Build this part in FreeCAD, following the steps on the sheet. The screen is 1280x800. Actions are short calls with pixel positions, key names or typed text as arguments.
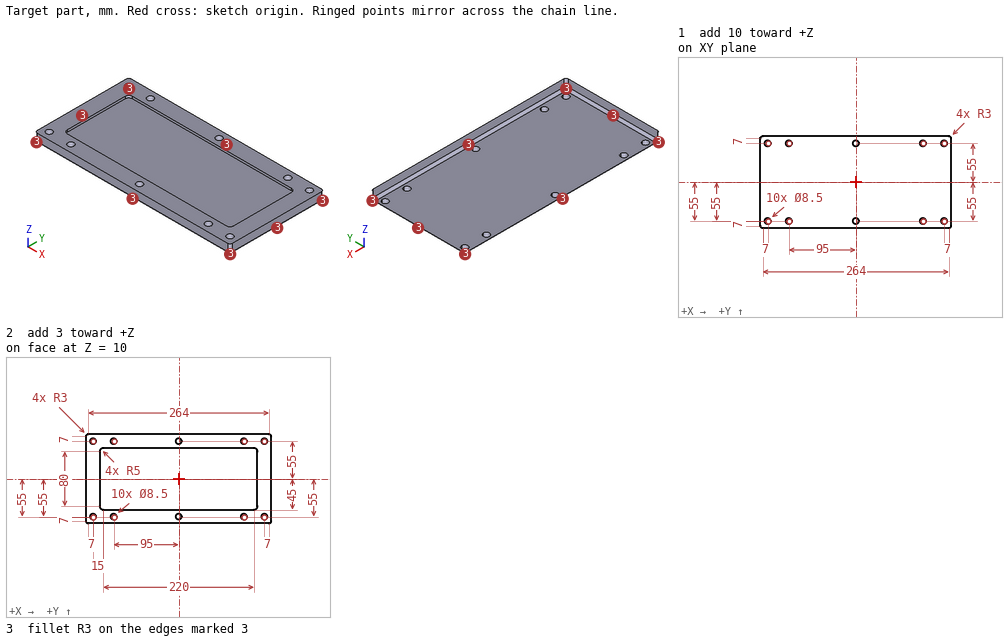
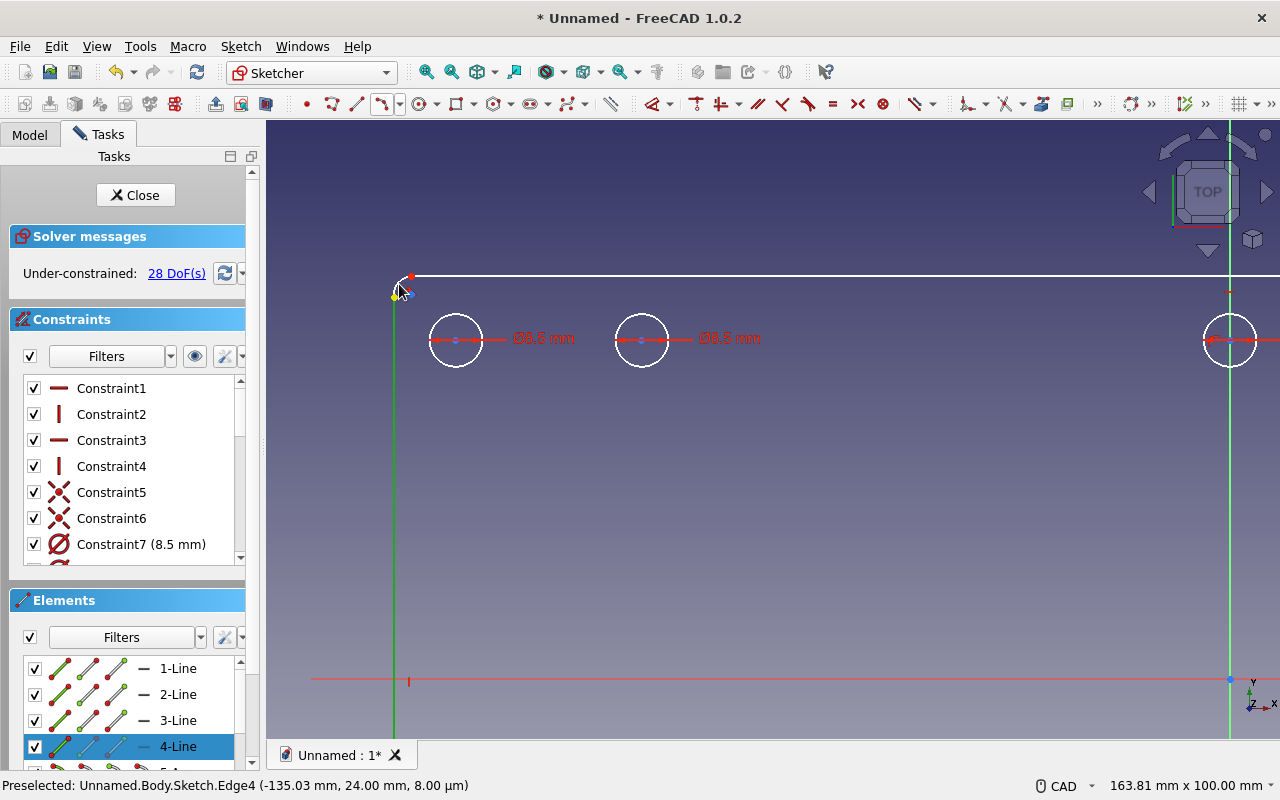
click(398, 283)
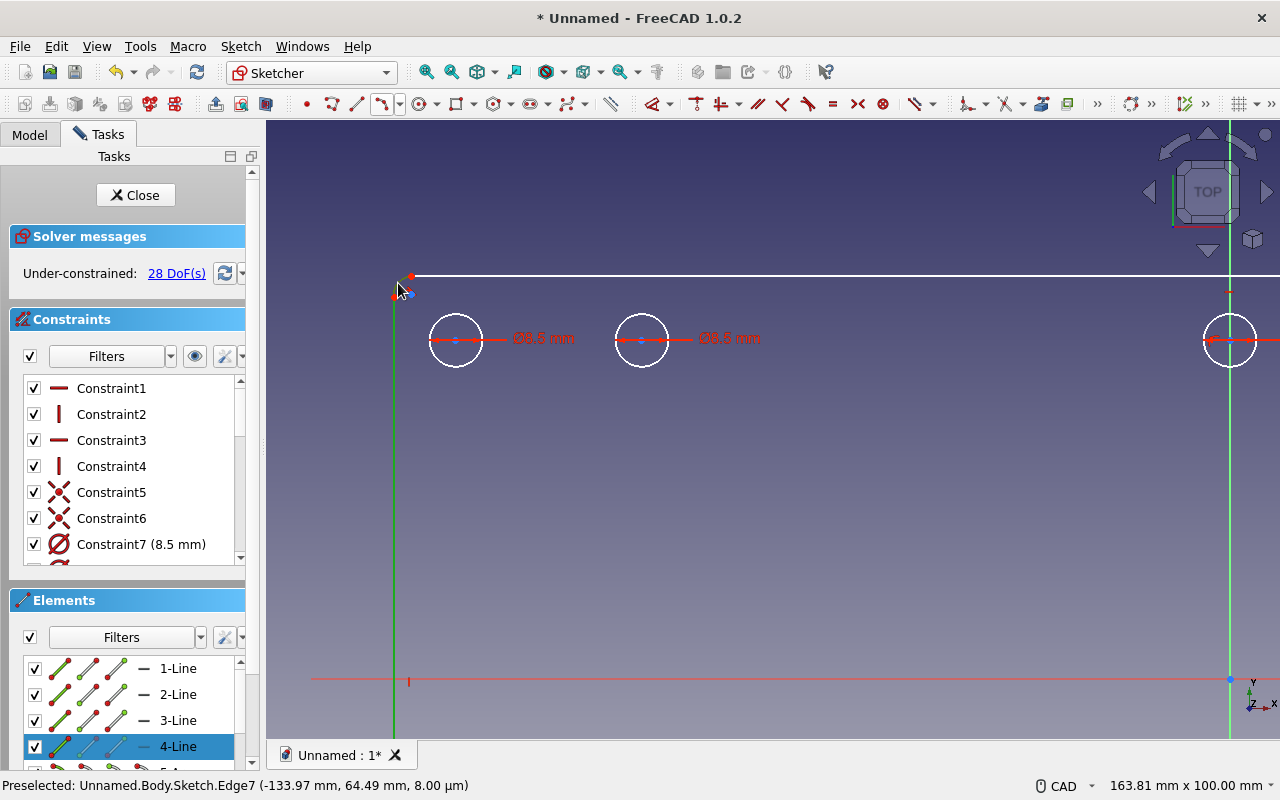
click(808, 104)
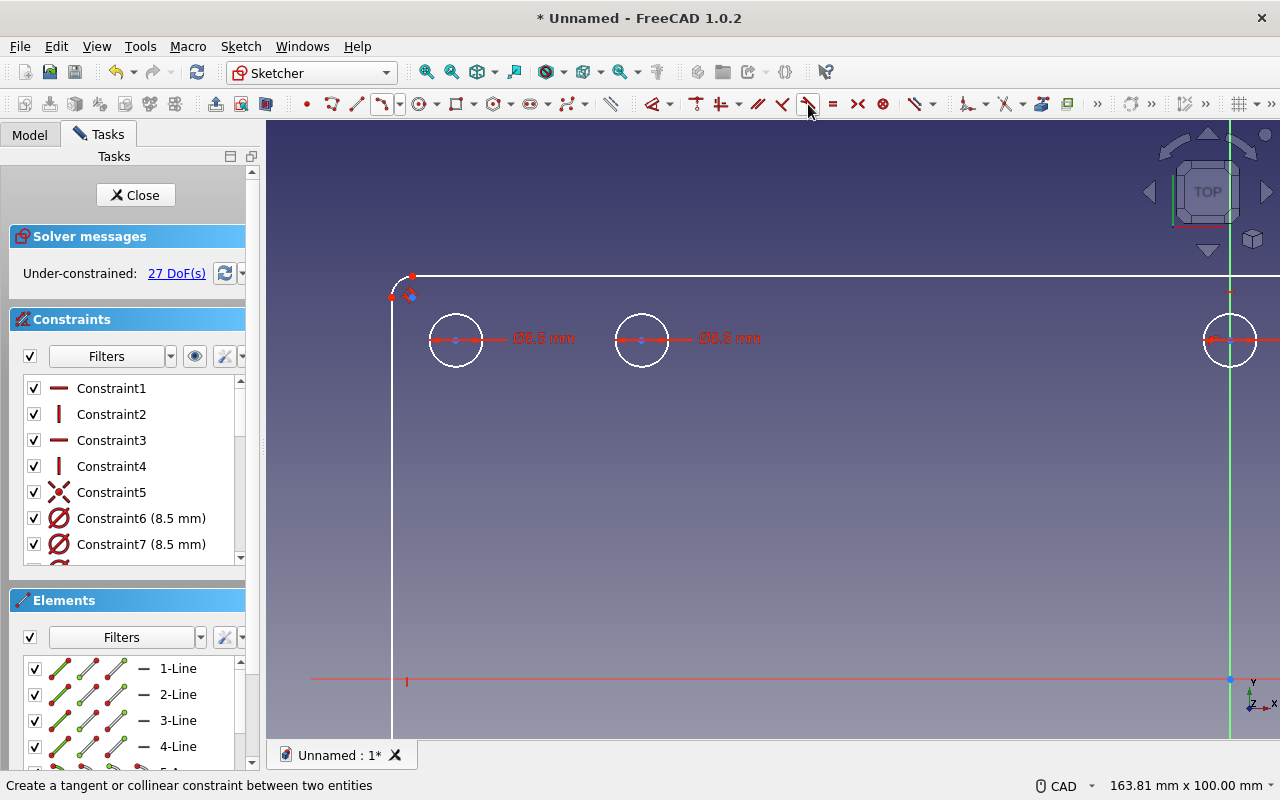
click(392, 528)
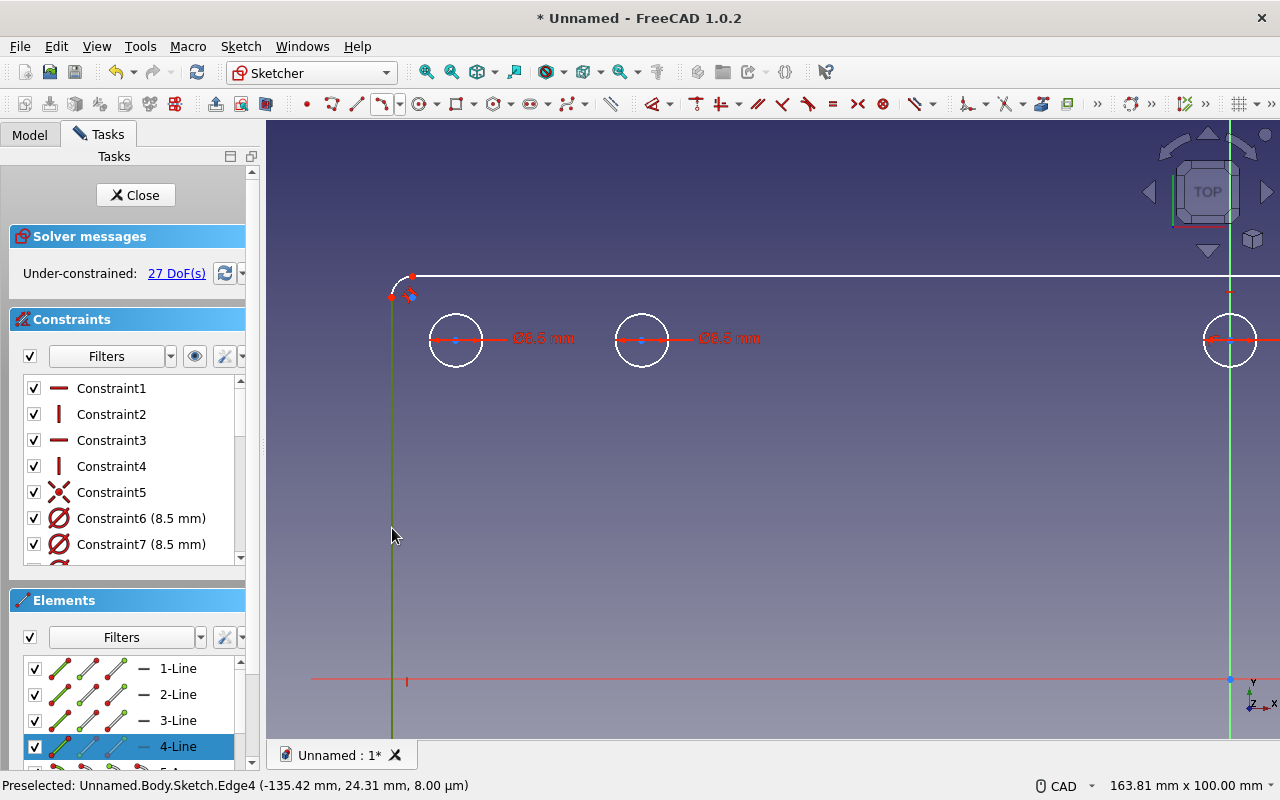
scroll(399, 284, down, 5)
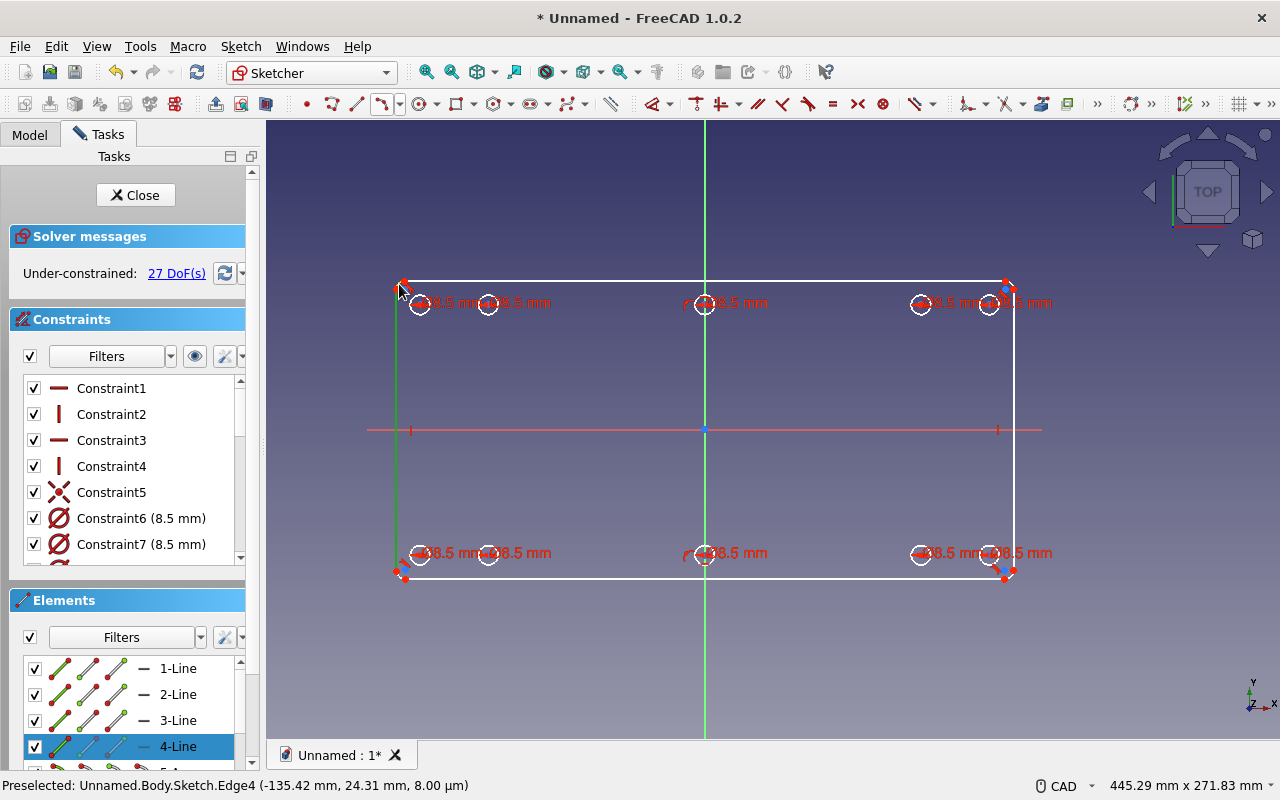
scroll(398, 575, up, 7)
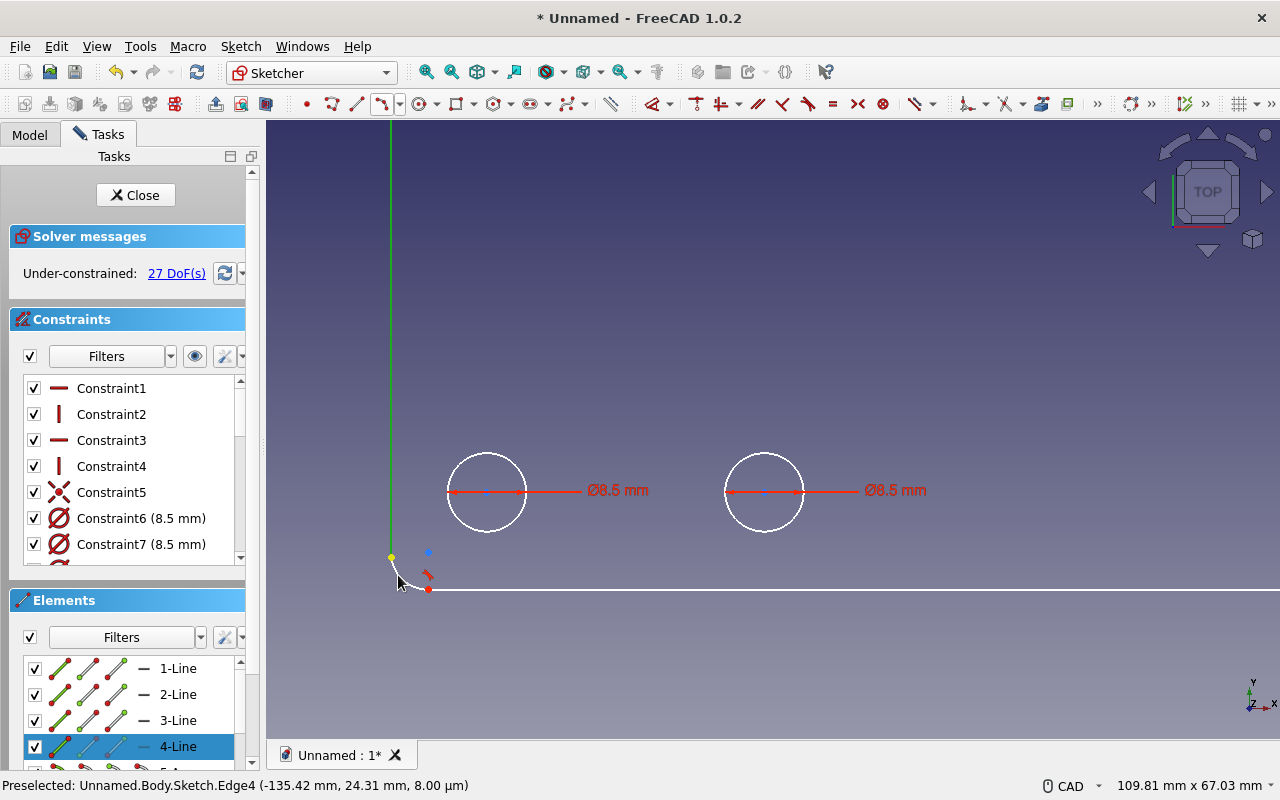
click(397, 573)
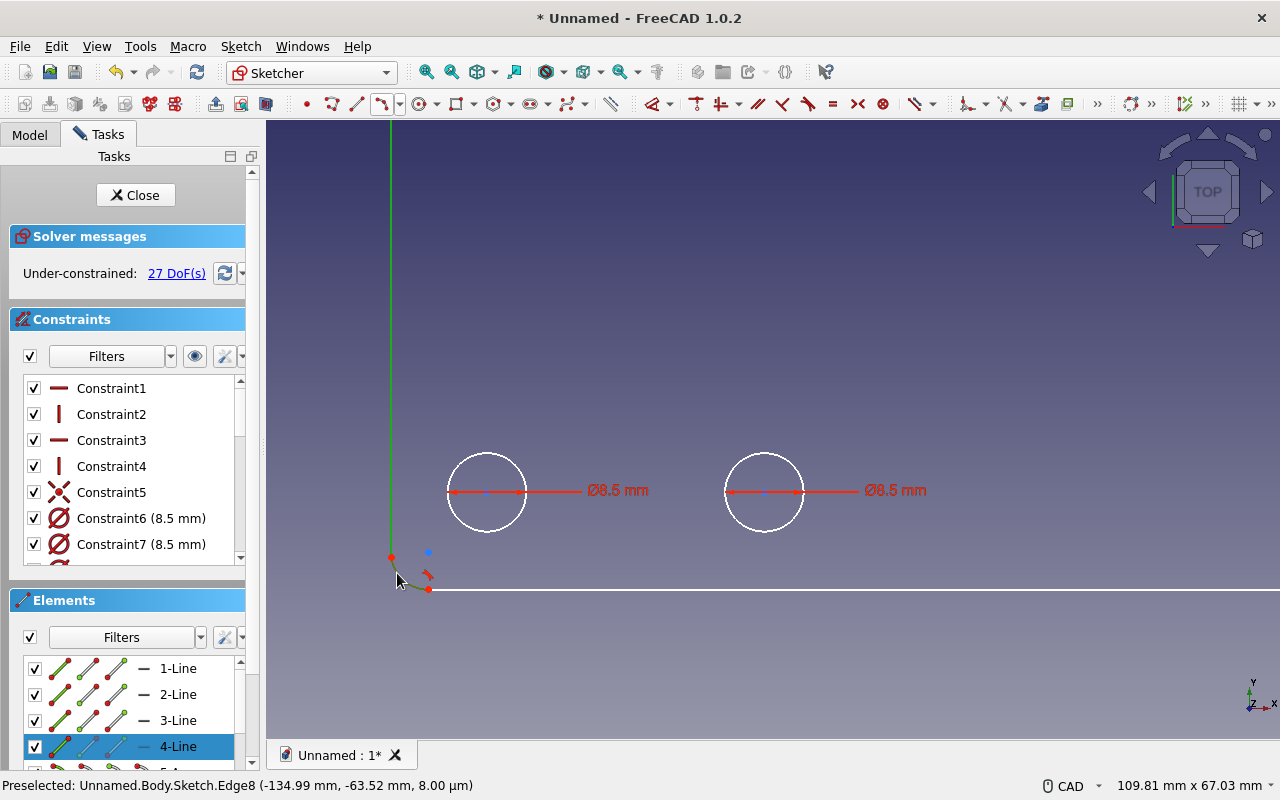
click(808, 104)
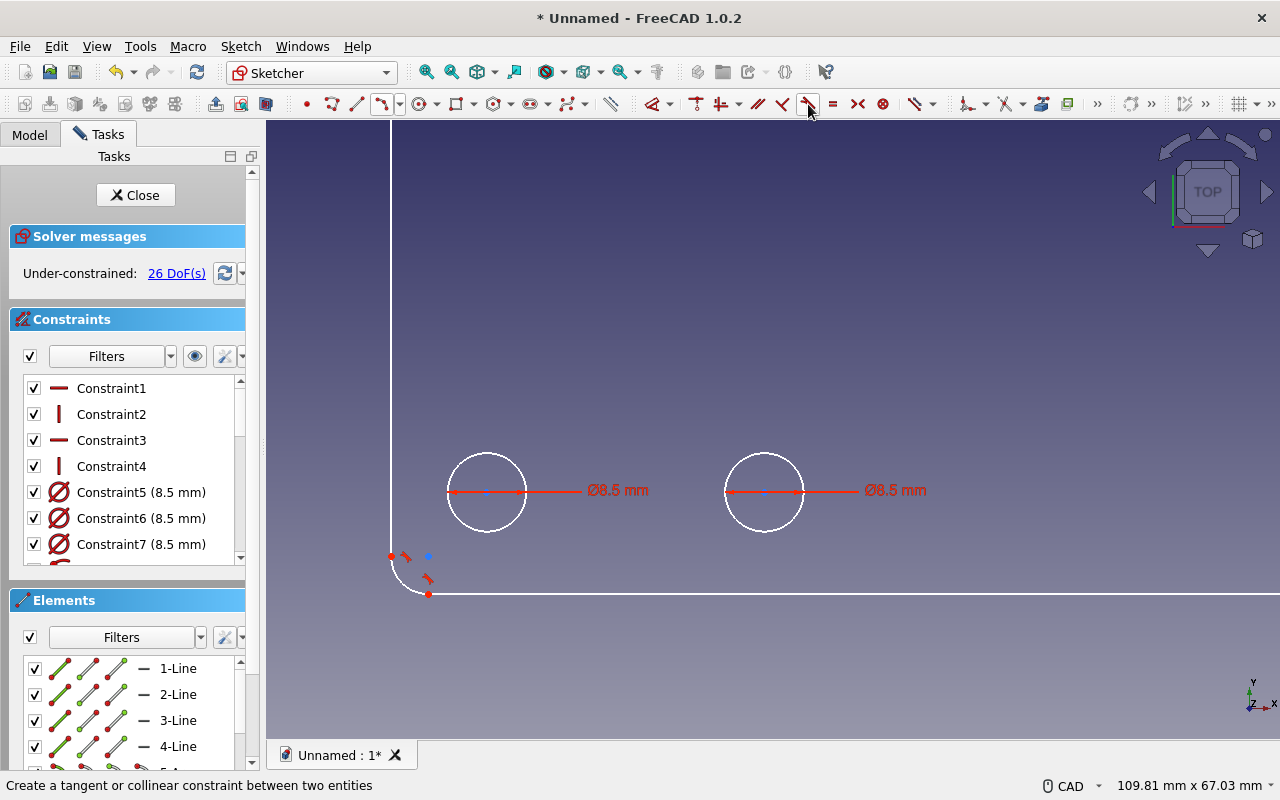
scroll(398, 576, down, 7)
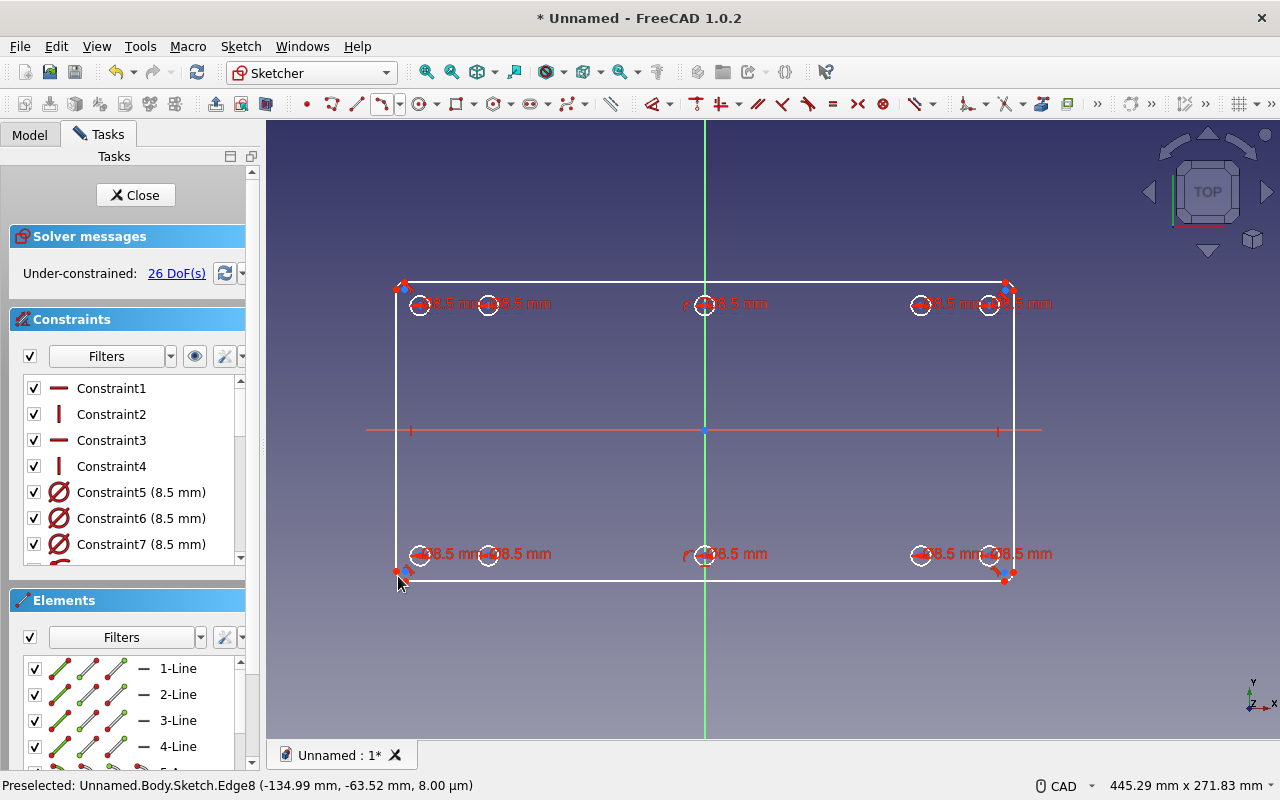
scroll(1009, 580, up, 7)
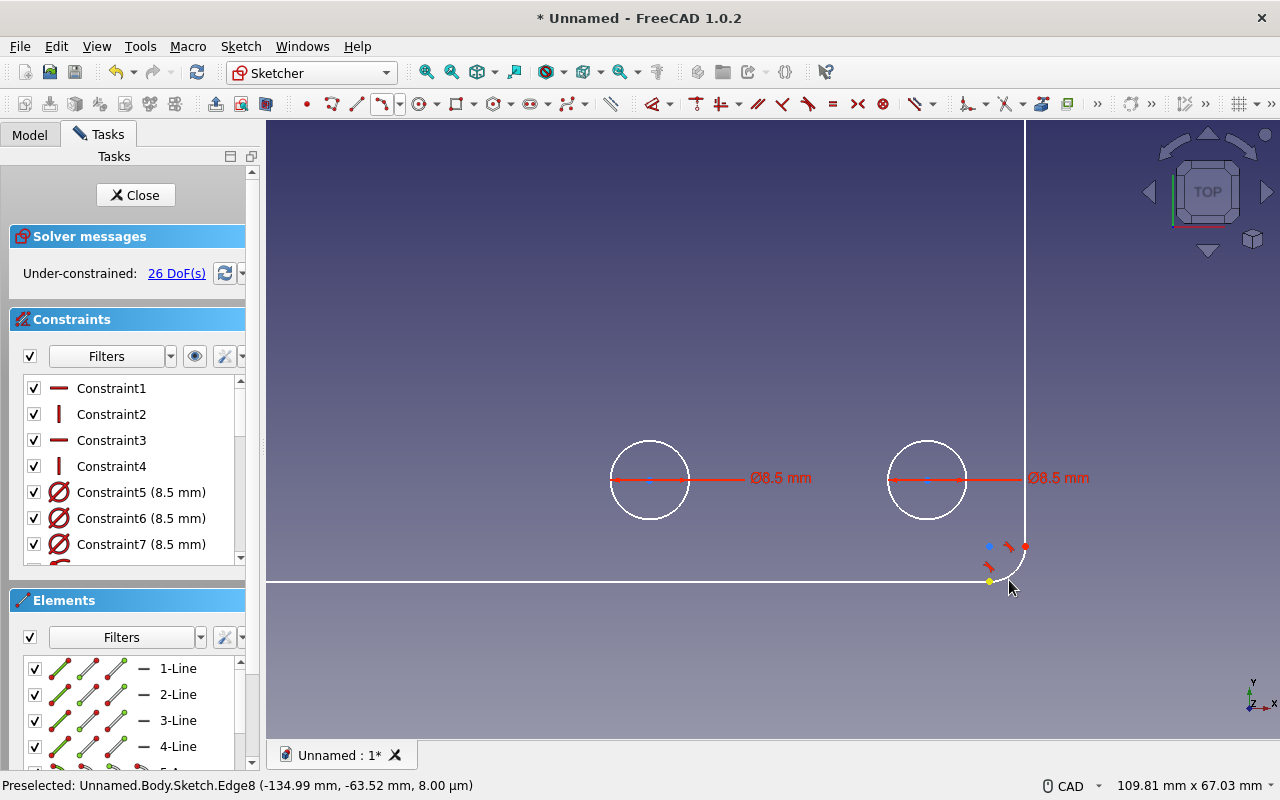
click(1006, 578)